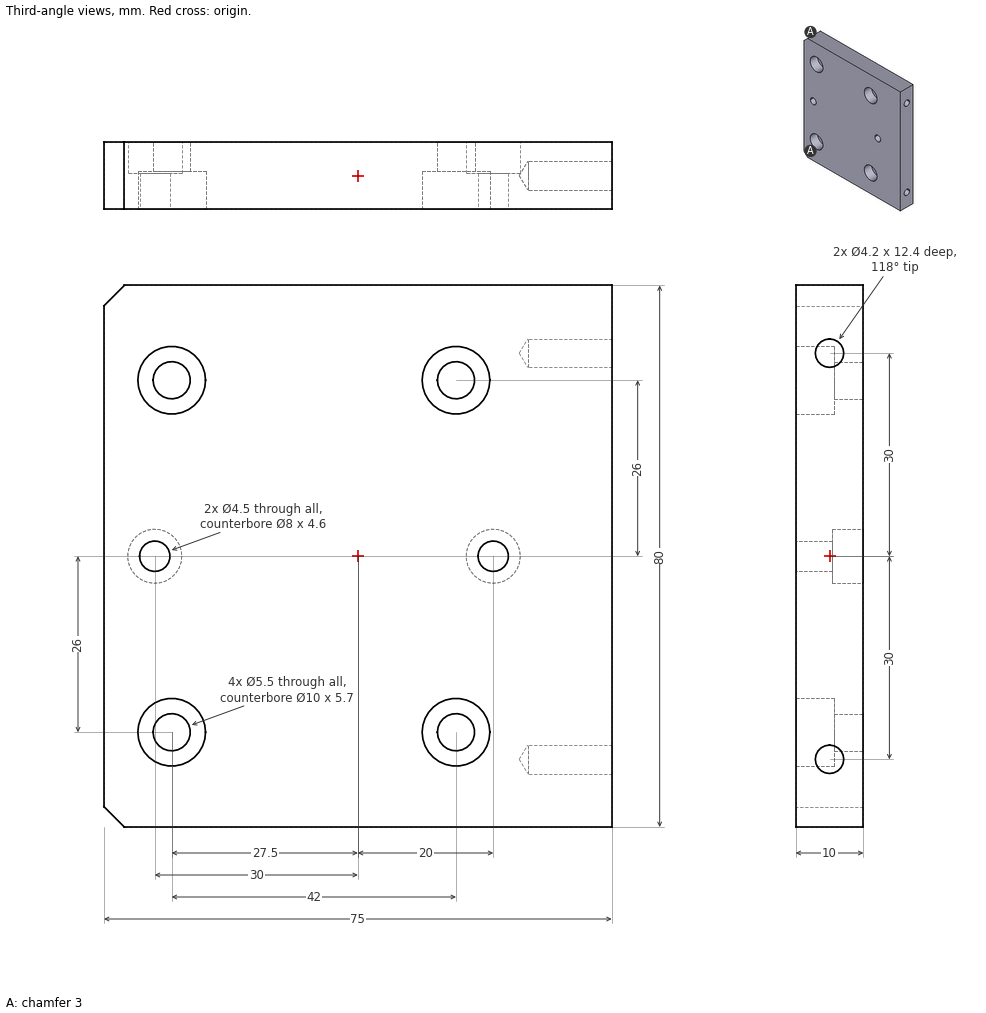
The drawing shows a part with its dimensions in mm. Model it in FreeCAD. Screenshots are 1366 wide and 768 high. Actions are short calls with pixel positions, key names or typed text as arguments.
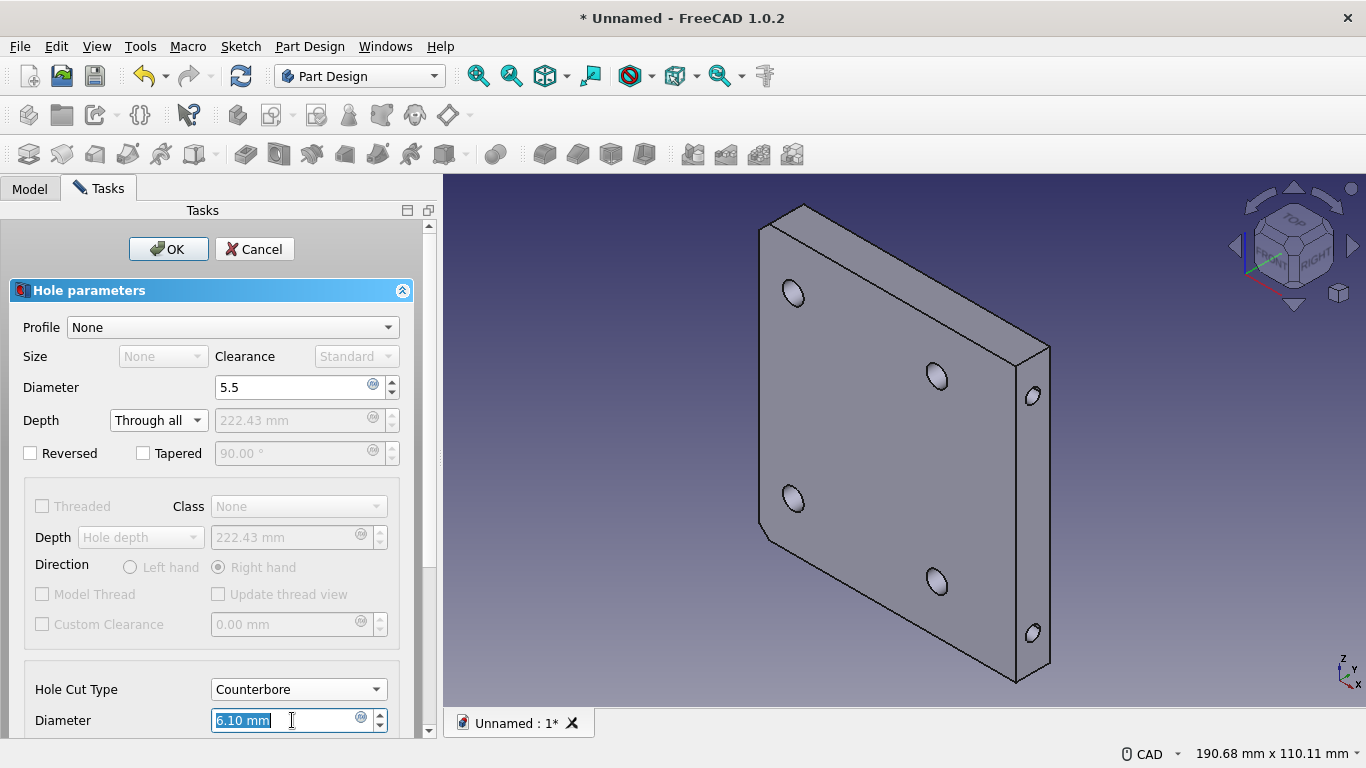
text(10)
key(Tab)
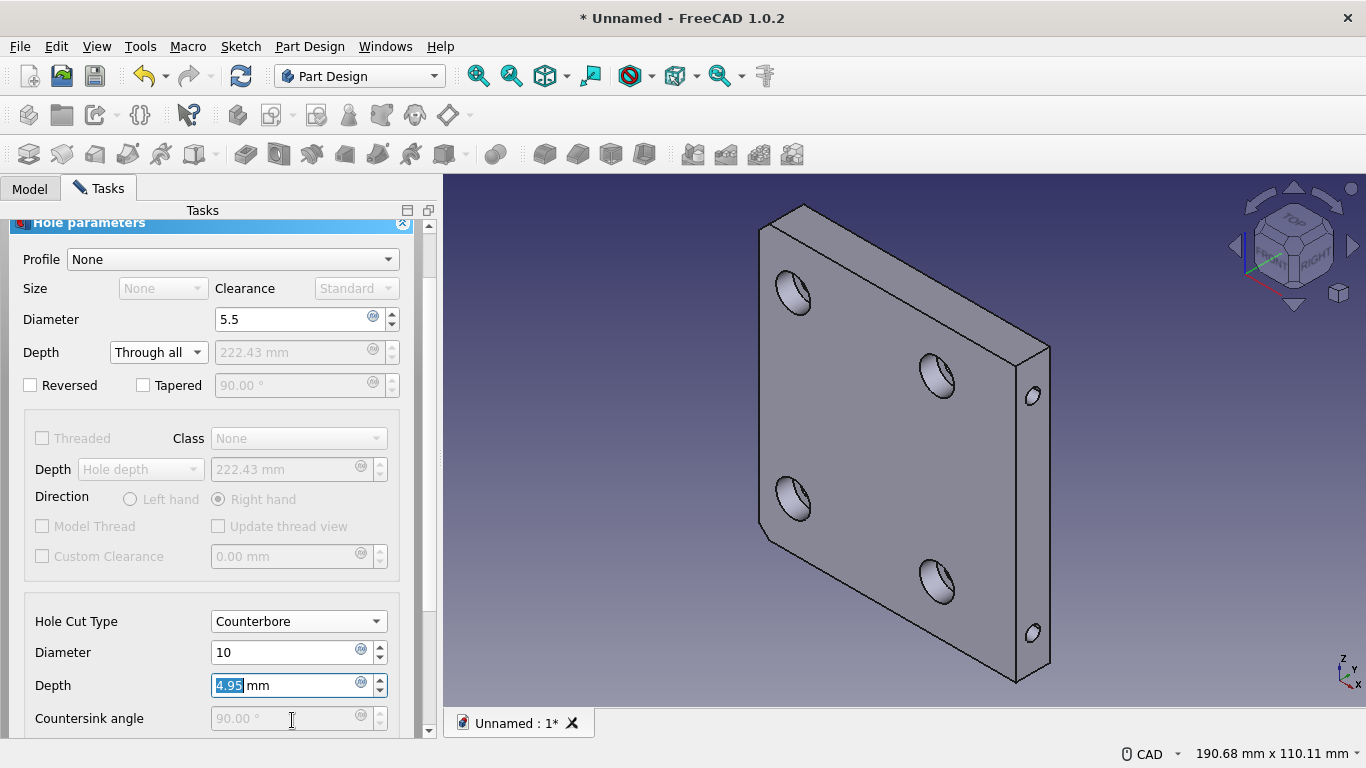
text(5.7)
key(Tab)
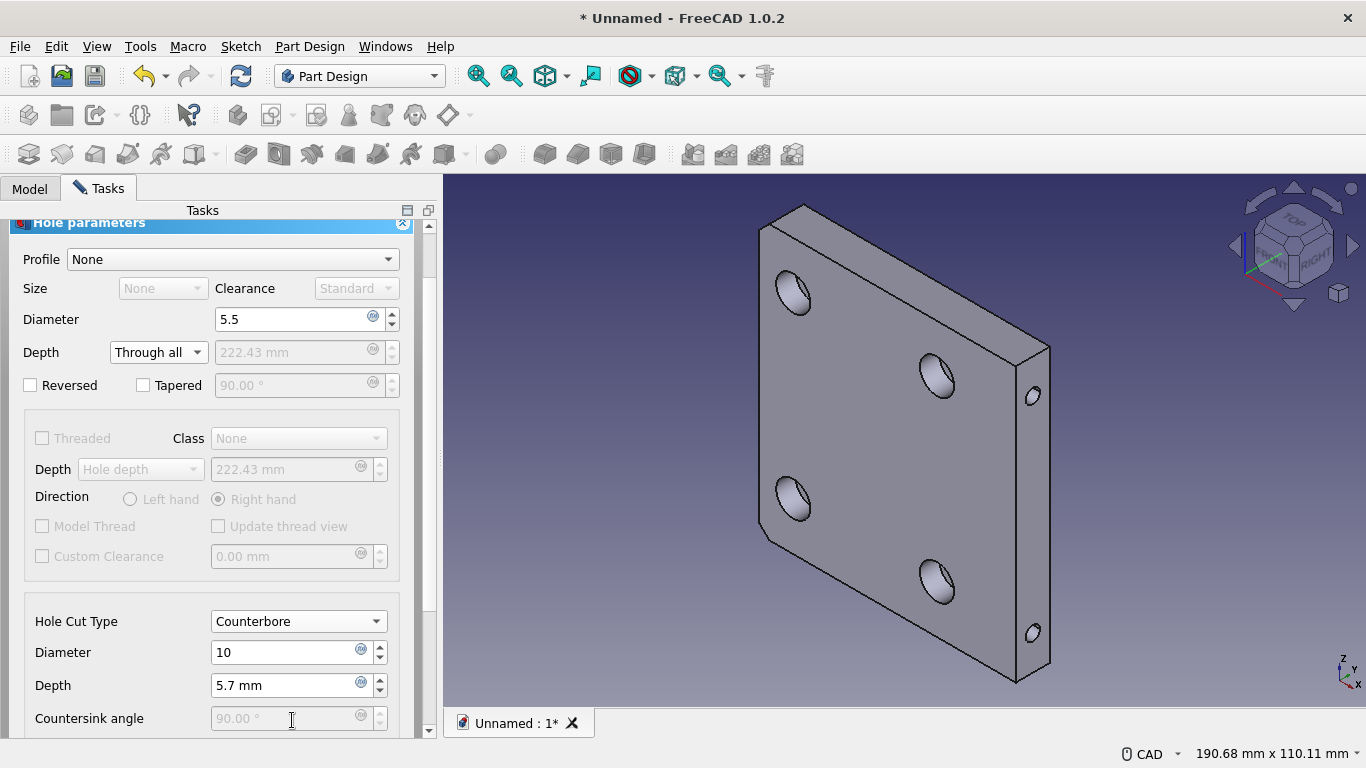
scroll(429, 479, up, 2)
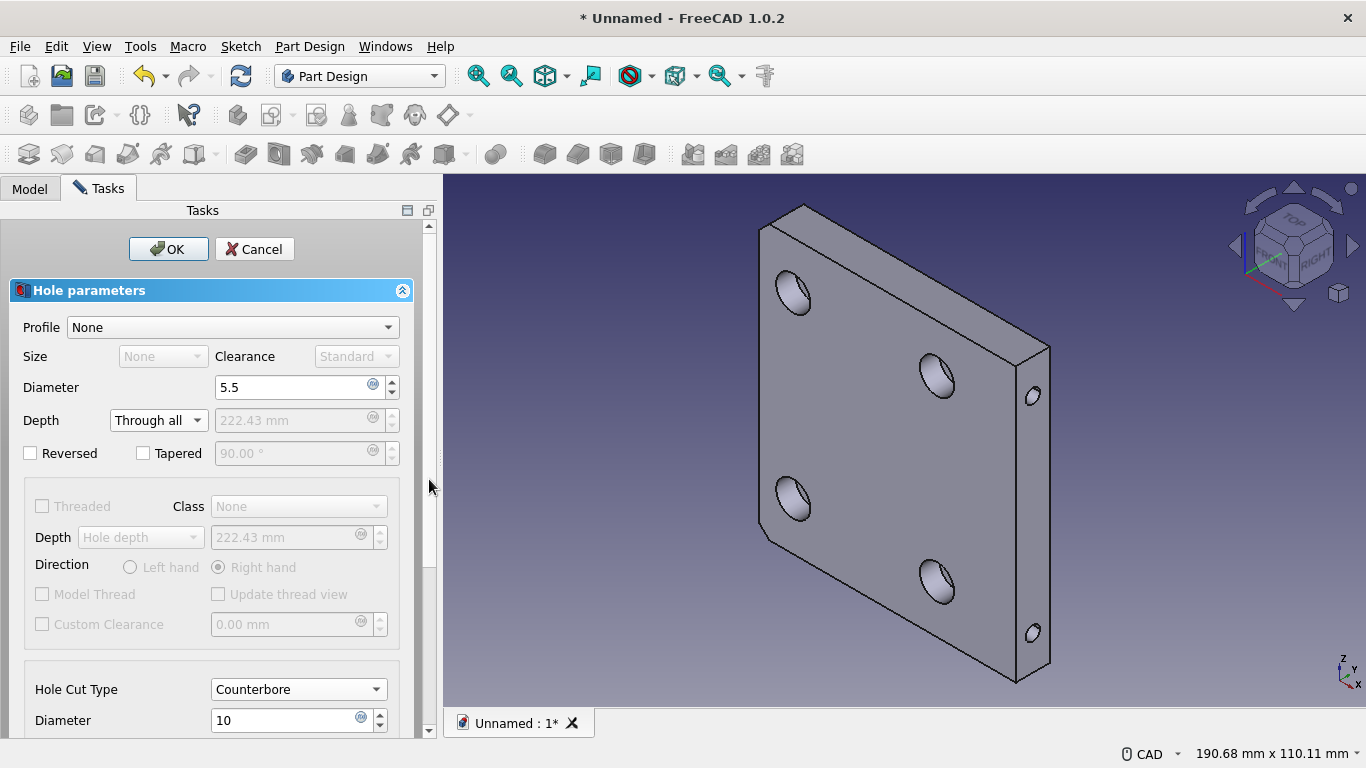
click(169, 249)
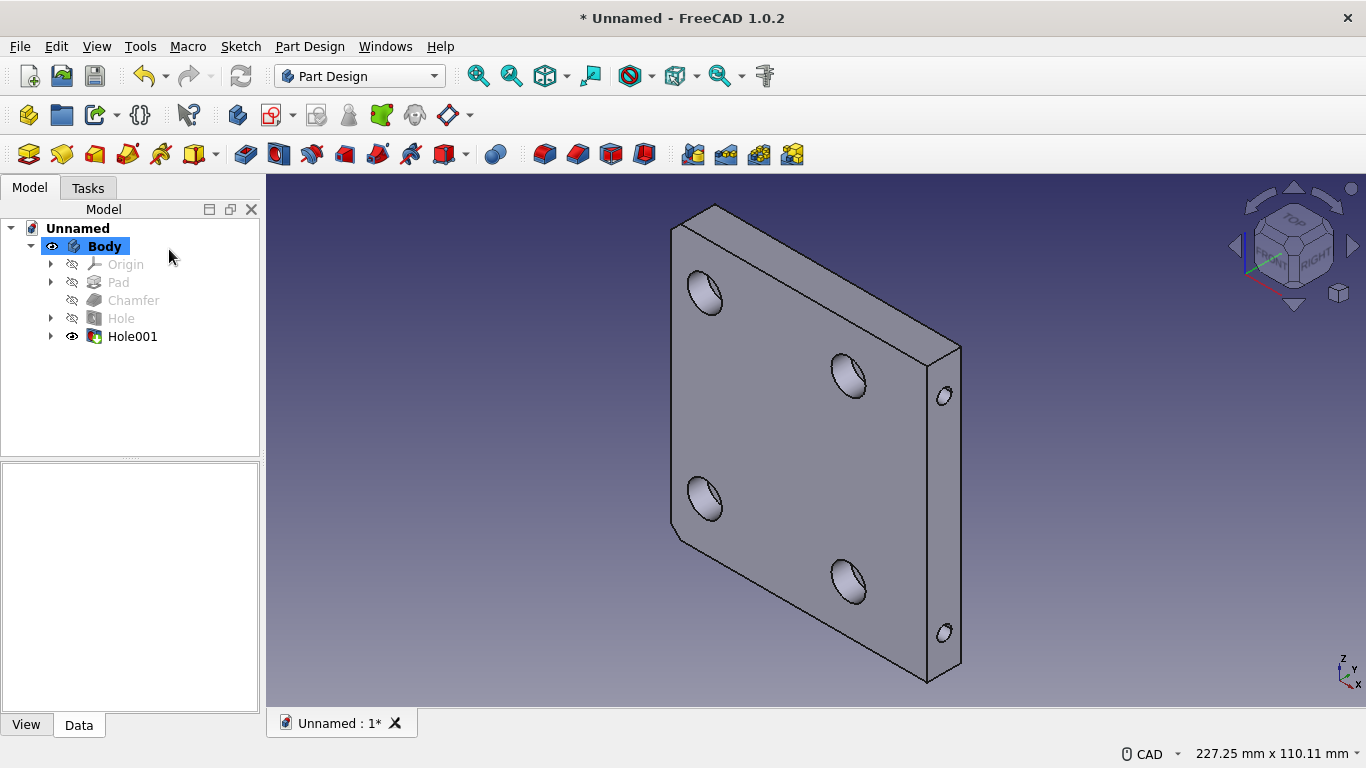
key(4)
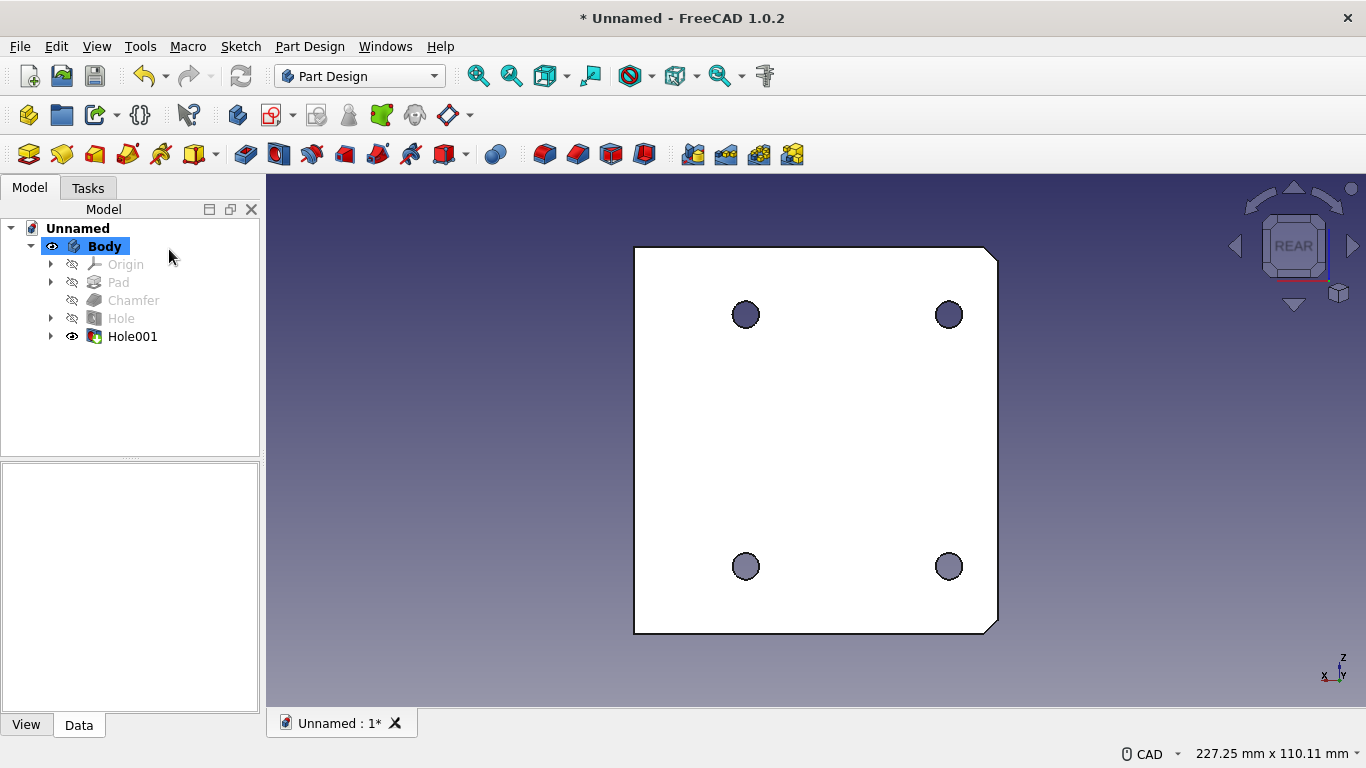
click(816, 440)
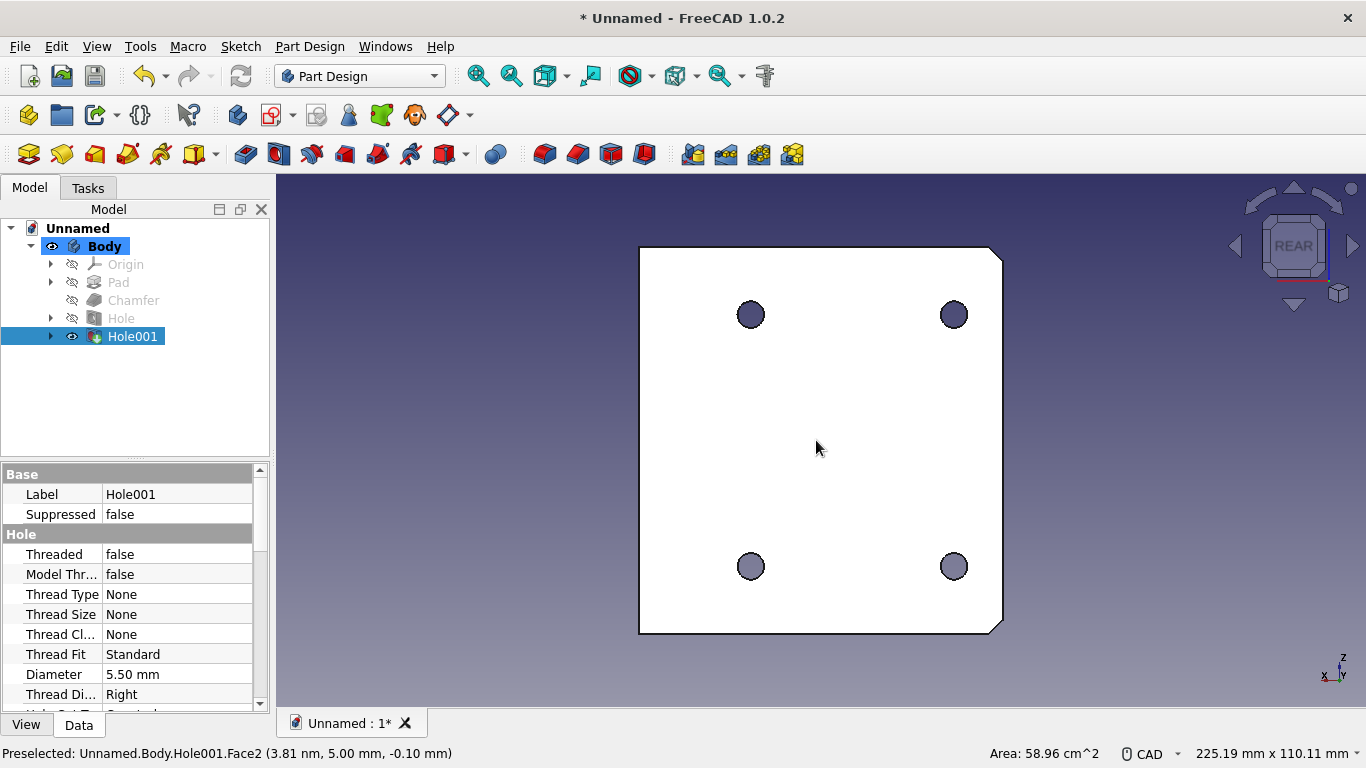
click(270, 116)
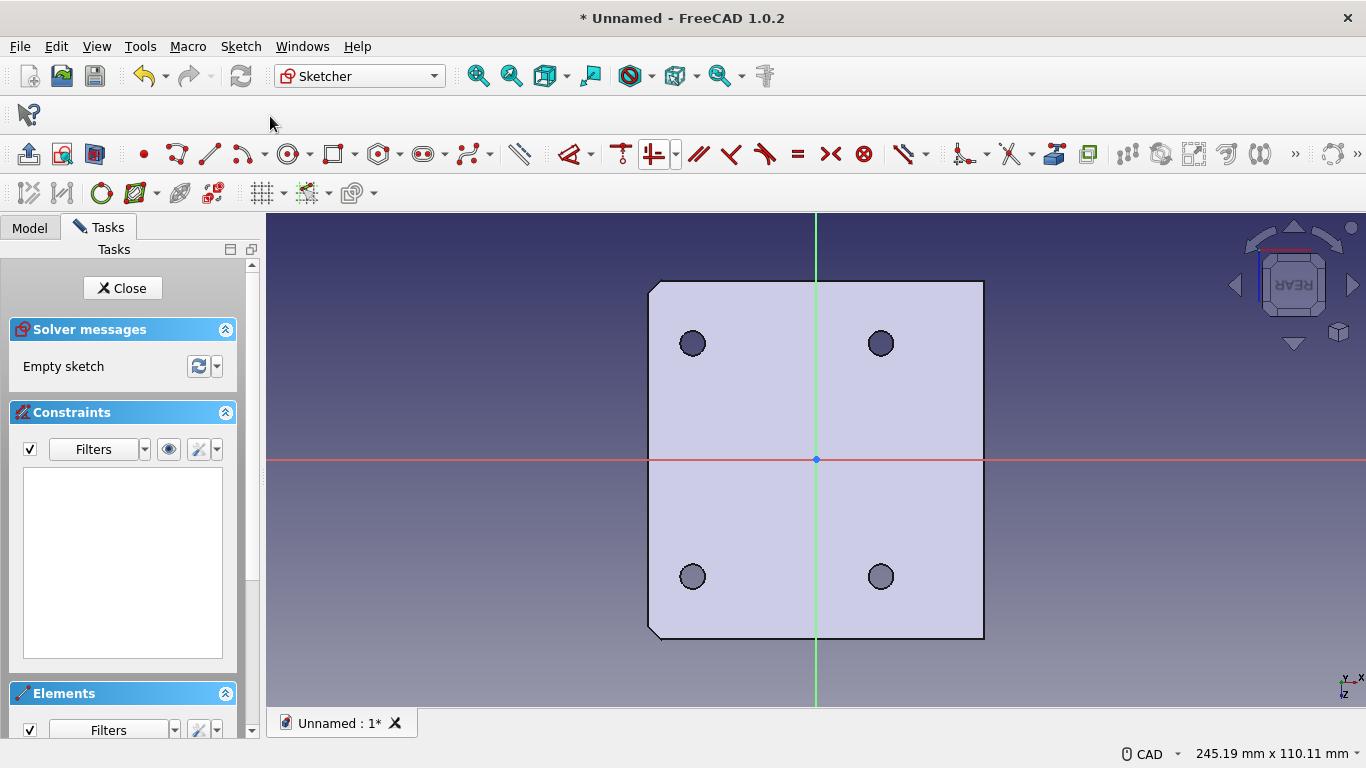
scroll(820, 460, up, 5)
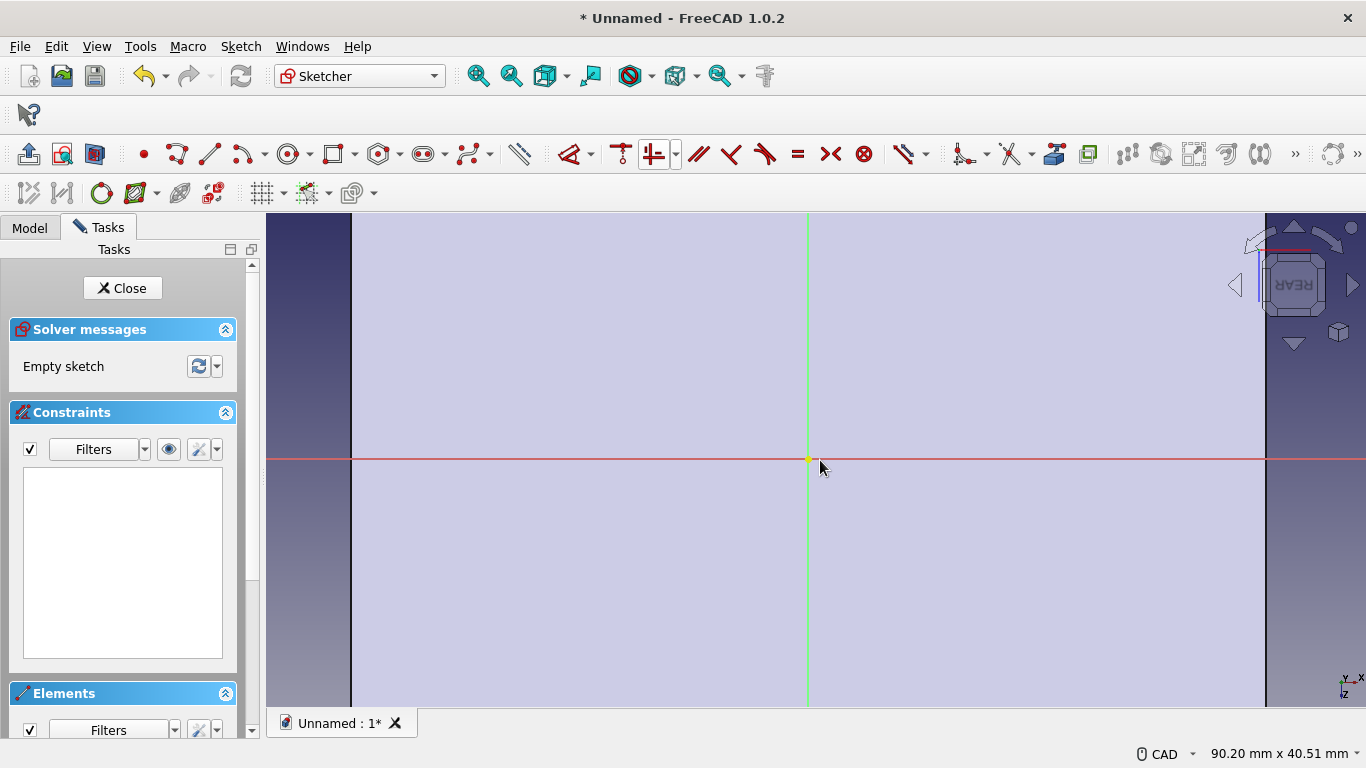
click(288, 154)